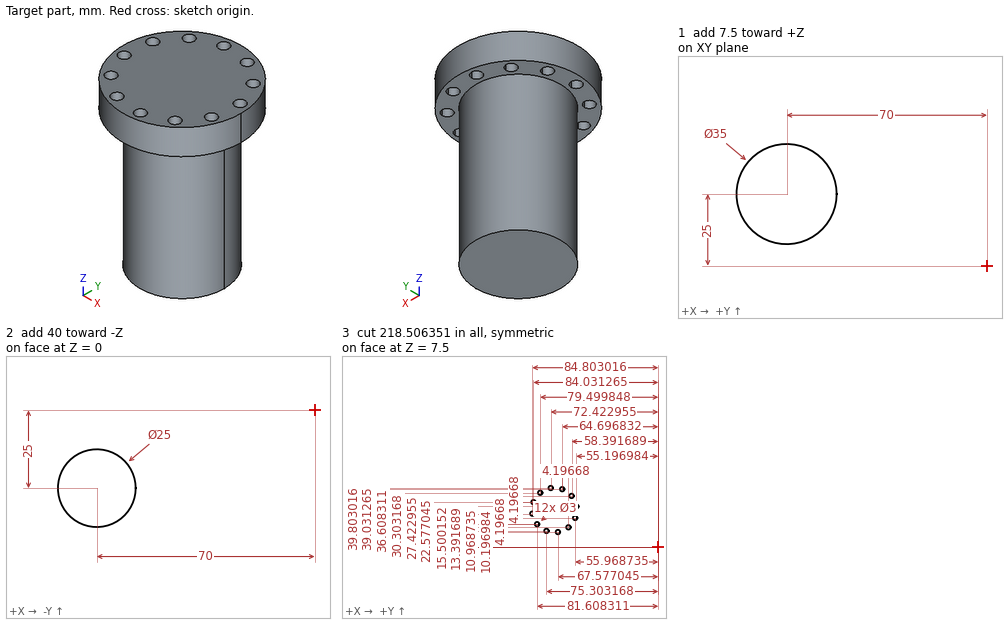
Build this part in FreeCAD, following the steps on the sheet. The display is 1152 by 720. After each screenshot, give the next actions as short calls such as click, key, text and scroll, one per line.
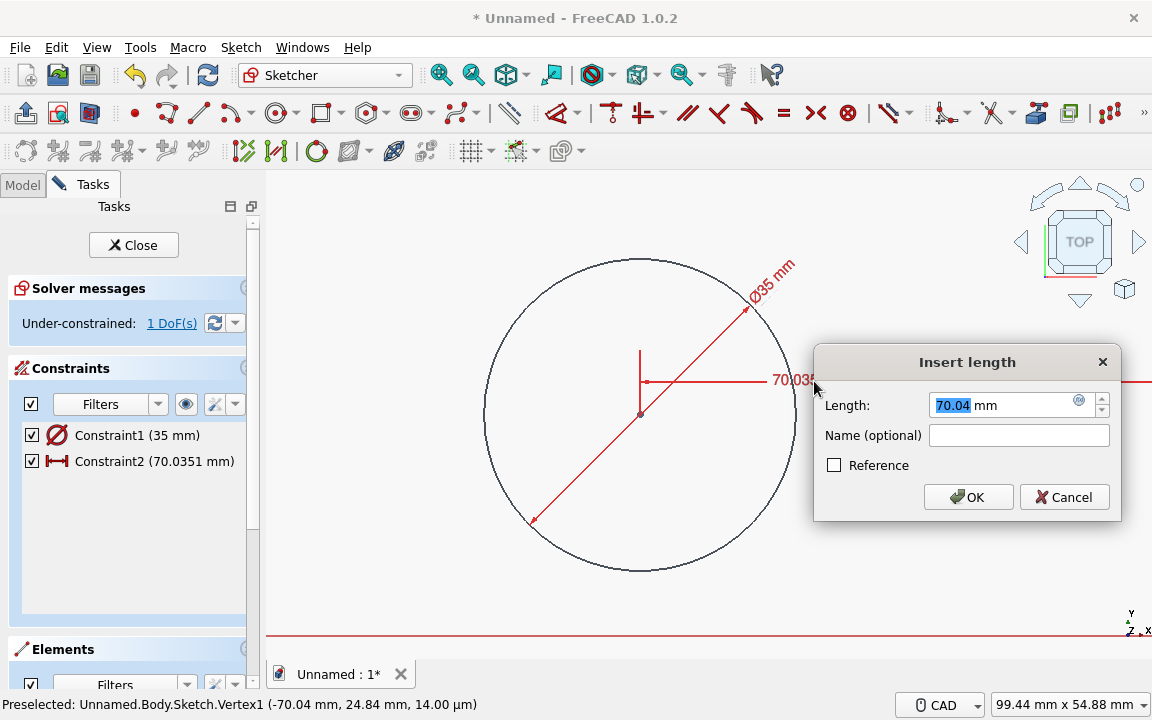
text(70)
key(Return)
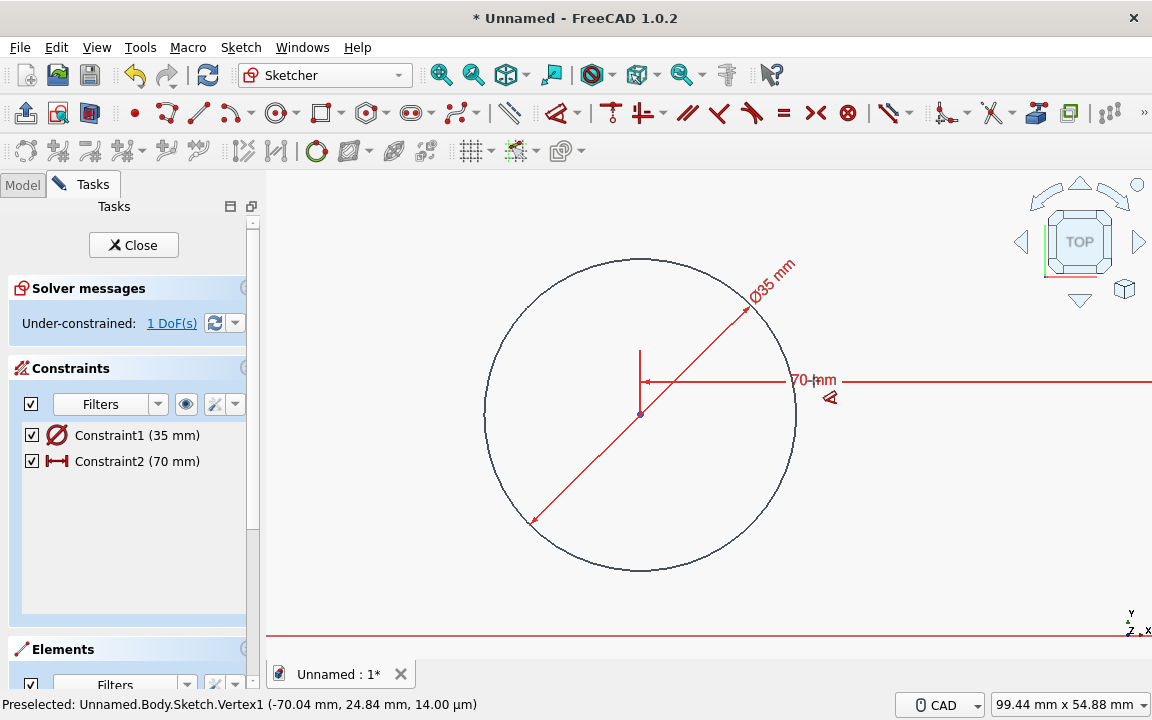
click(640, 415)
click(606, 523)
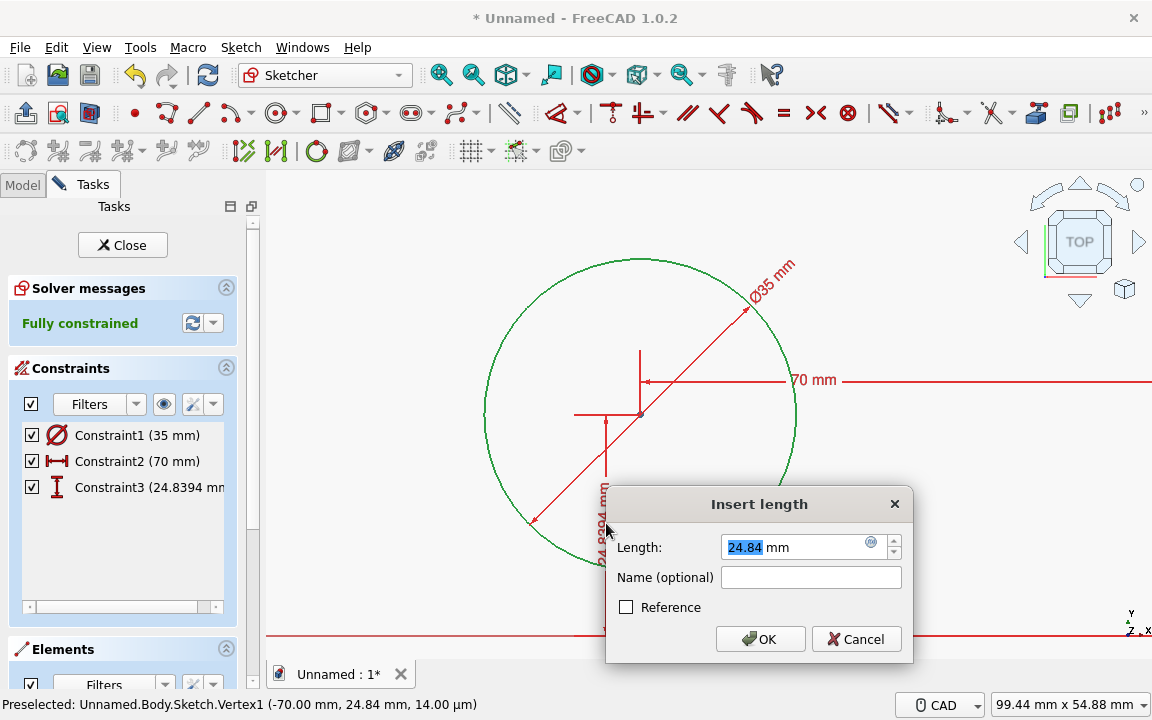
text(25)
key(Return)
key(Escape)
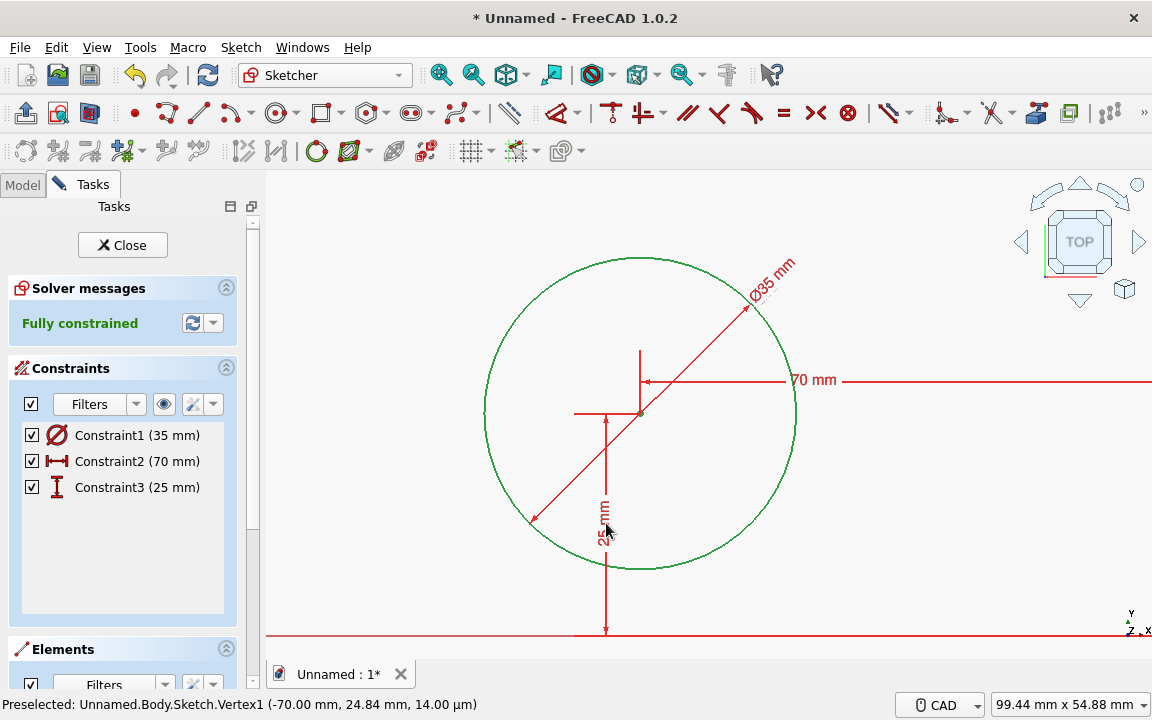
click(123, 245)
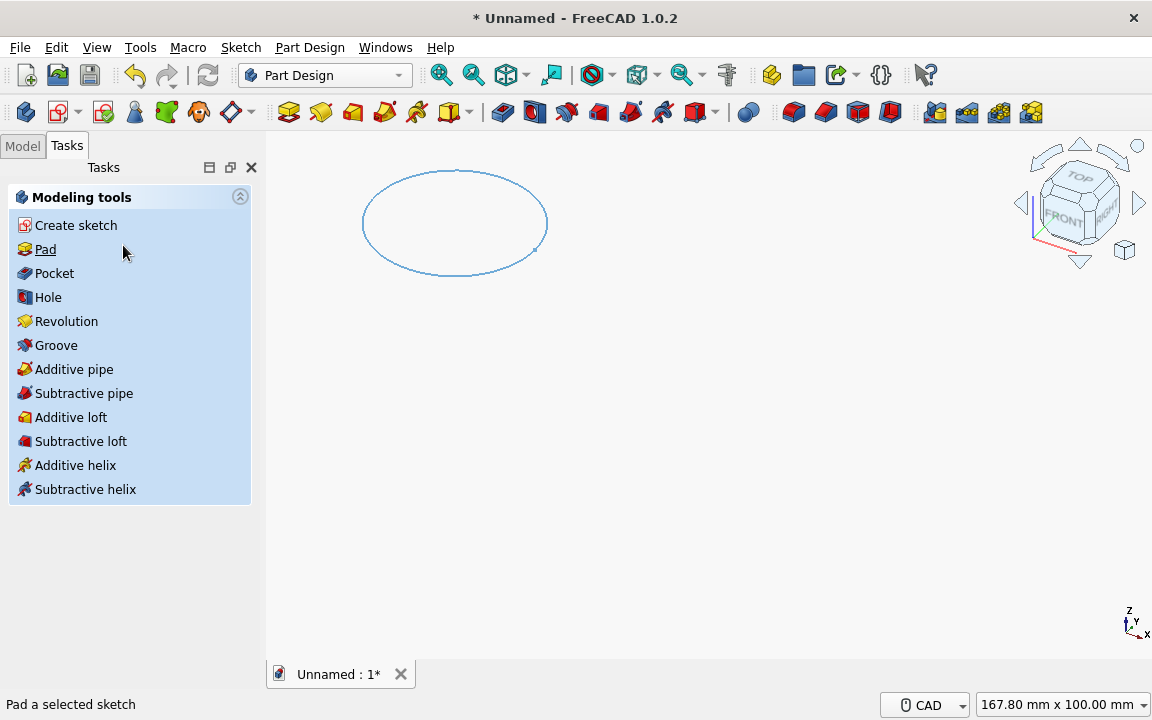
click(290, 112)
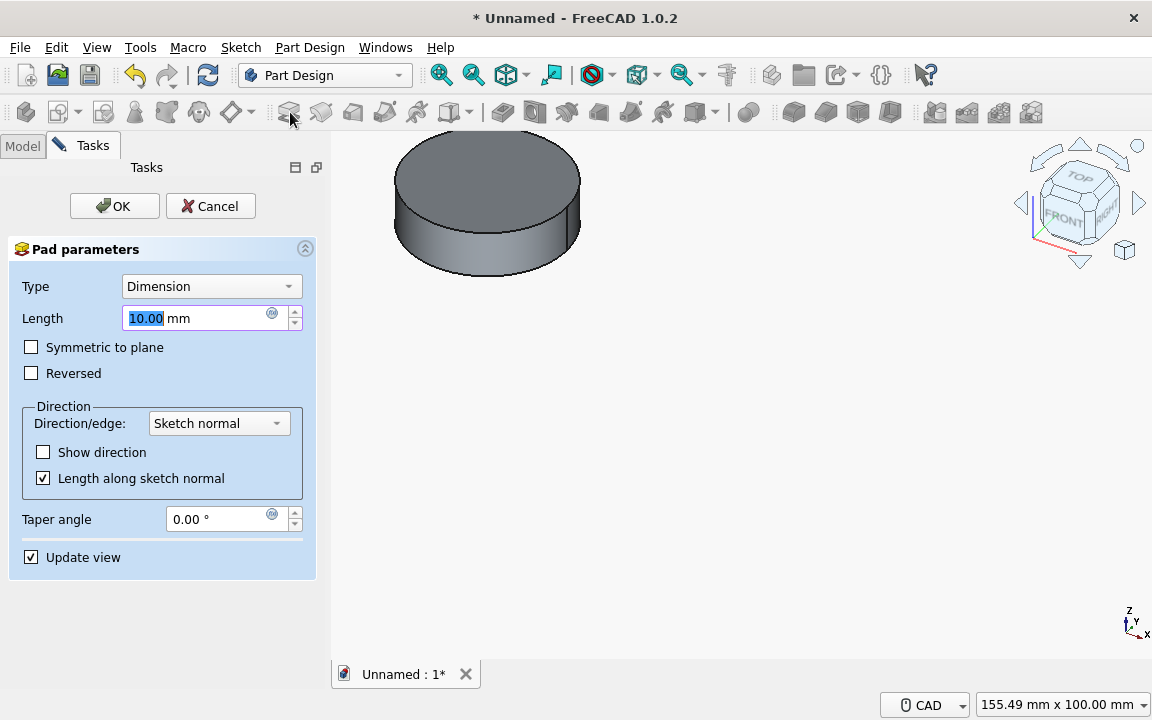
text(7.5)
key(Tab)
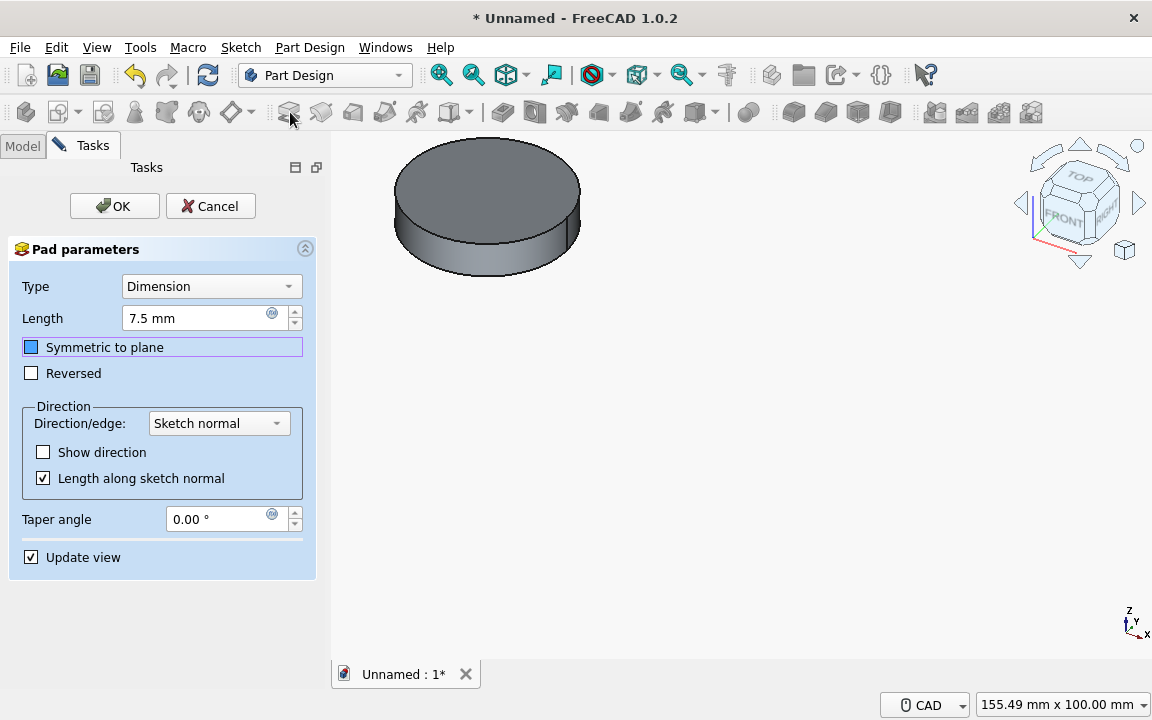
click(115, 206)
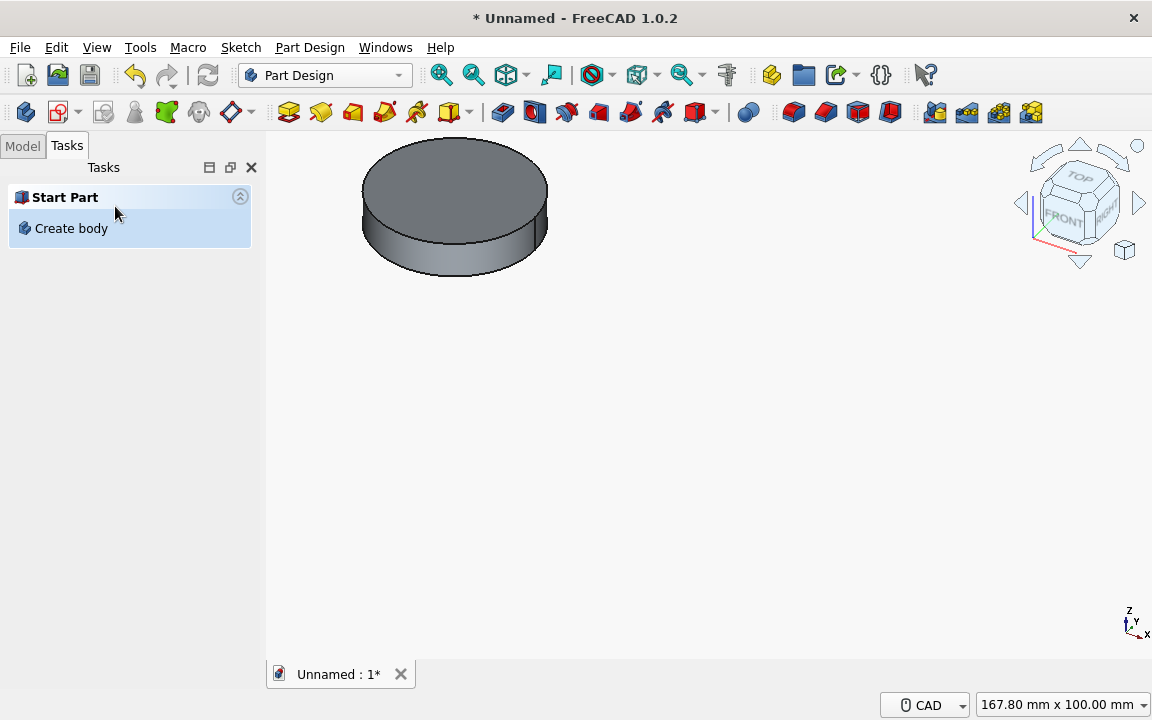
key(v)
key(f)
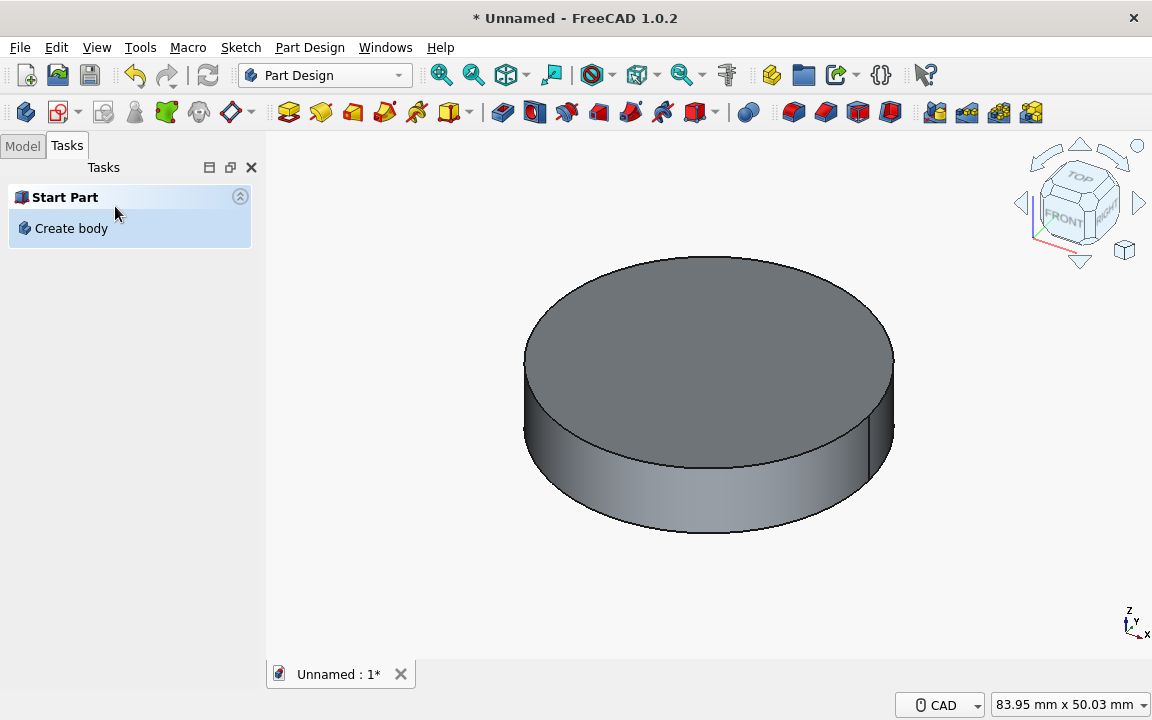
key(5)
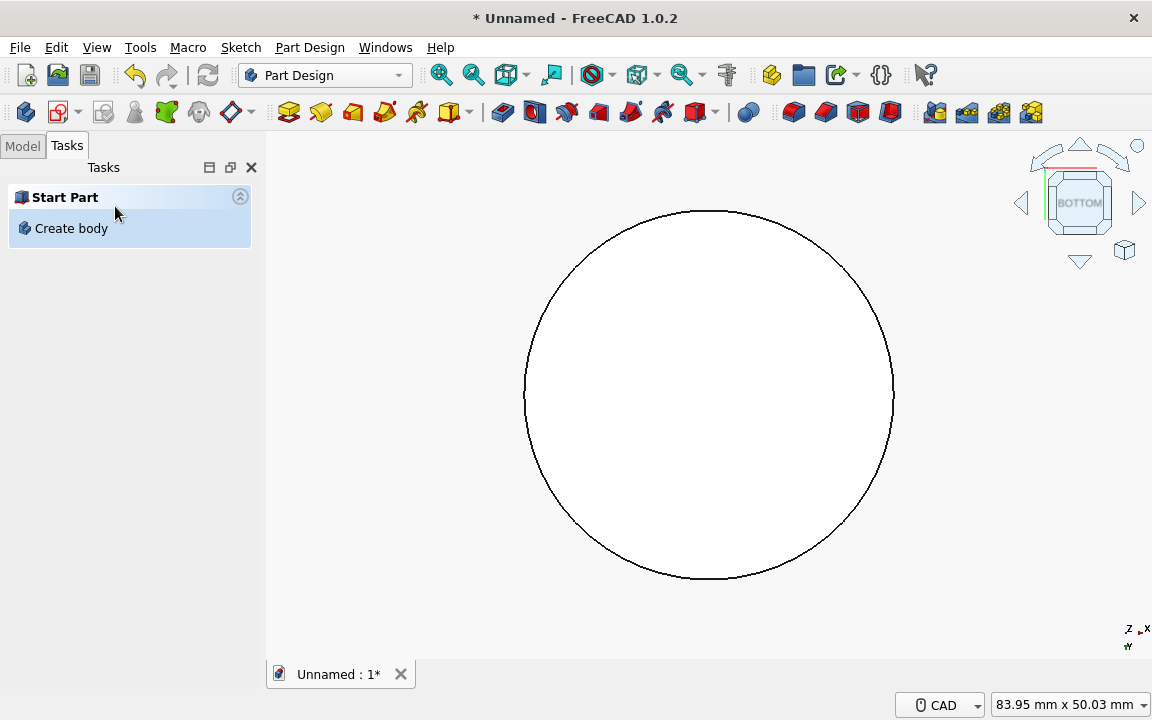
click(709, 394)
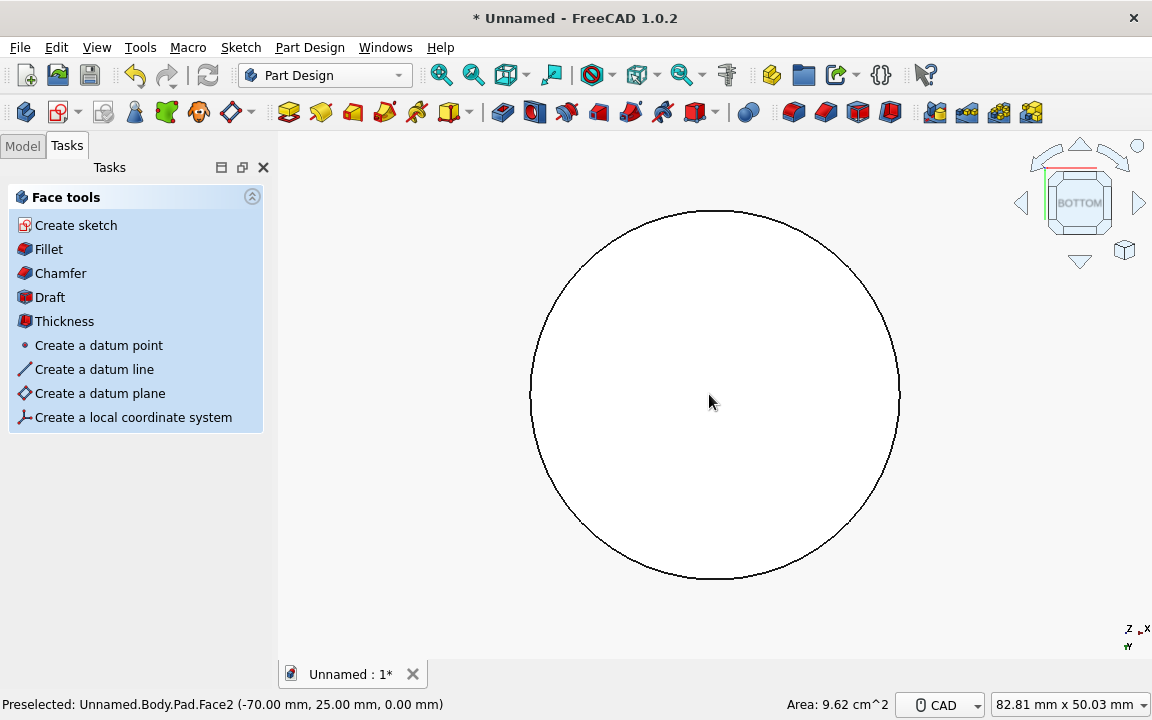
click(58, 112)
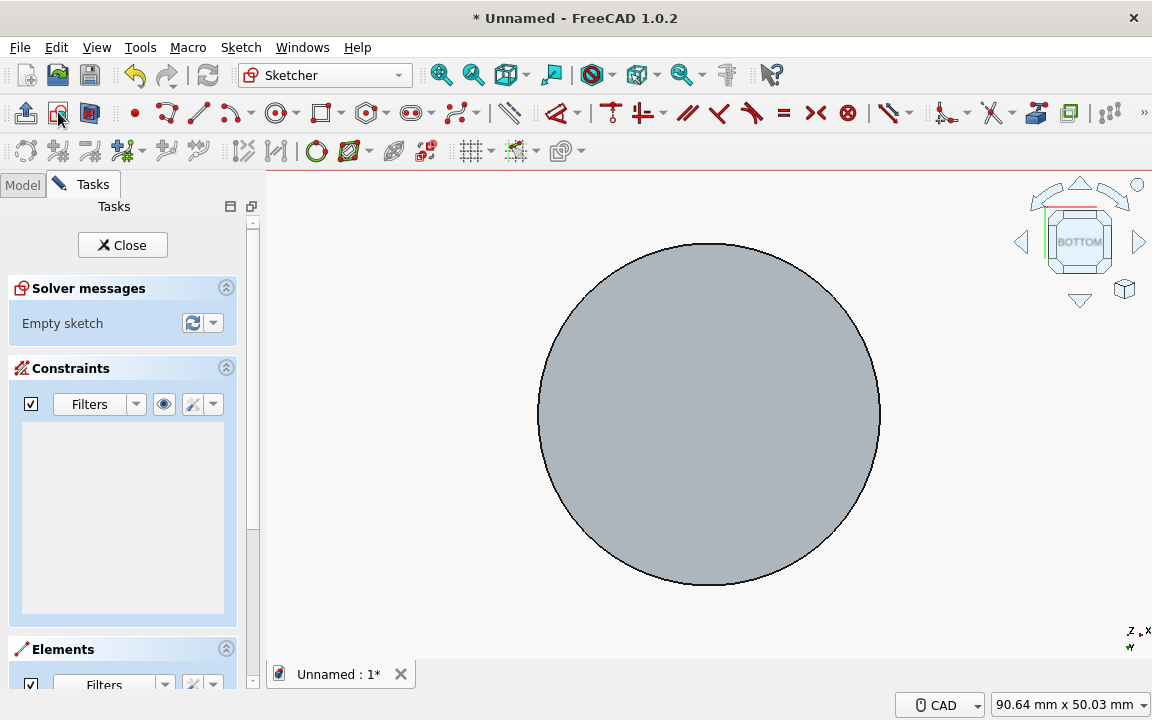
click(276, 114)